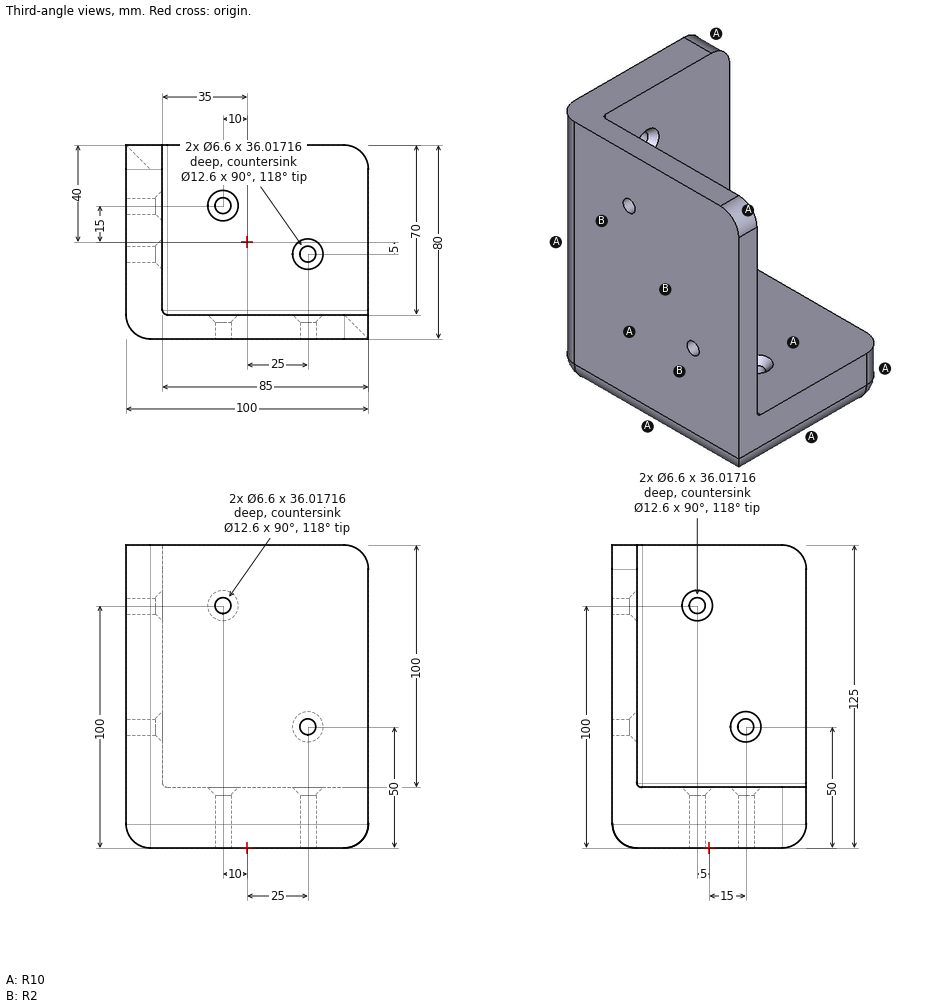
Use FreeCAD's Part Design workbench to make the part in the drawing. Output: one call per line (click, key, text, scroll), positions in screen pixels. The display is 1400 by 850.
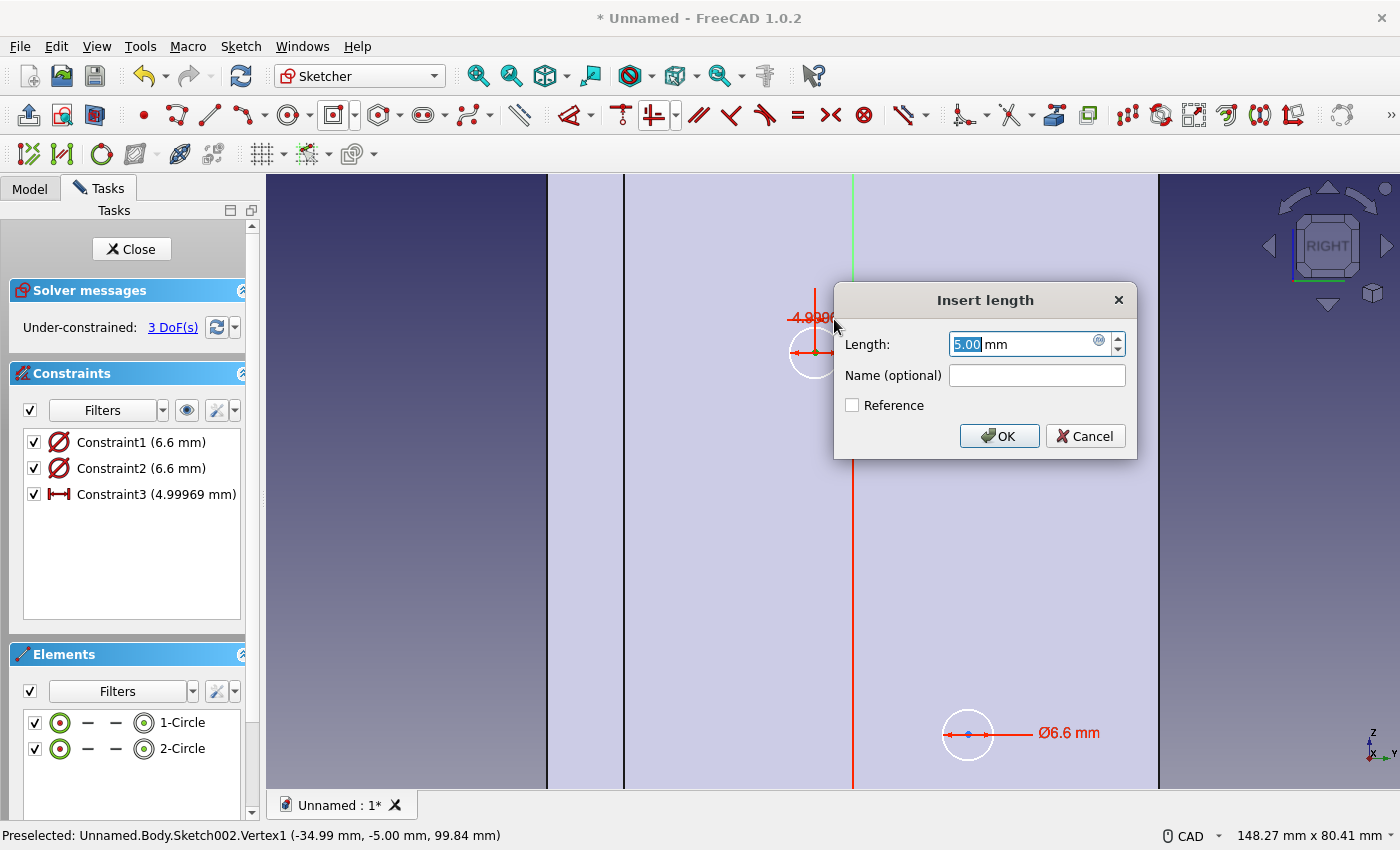
text(5)
key(Return)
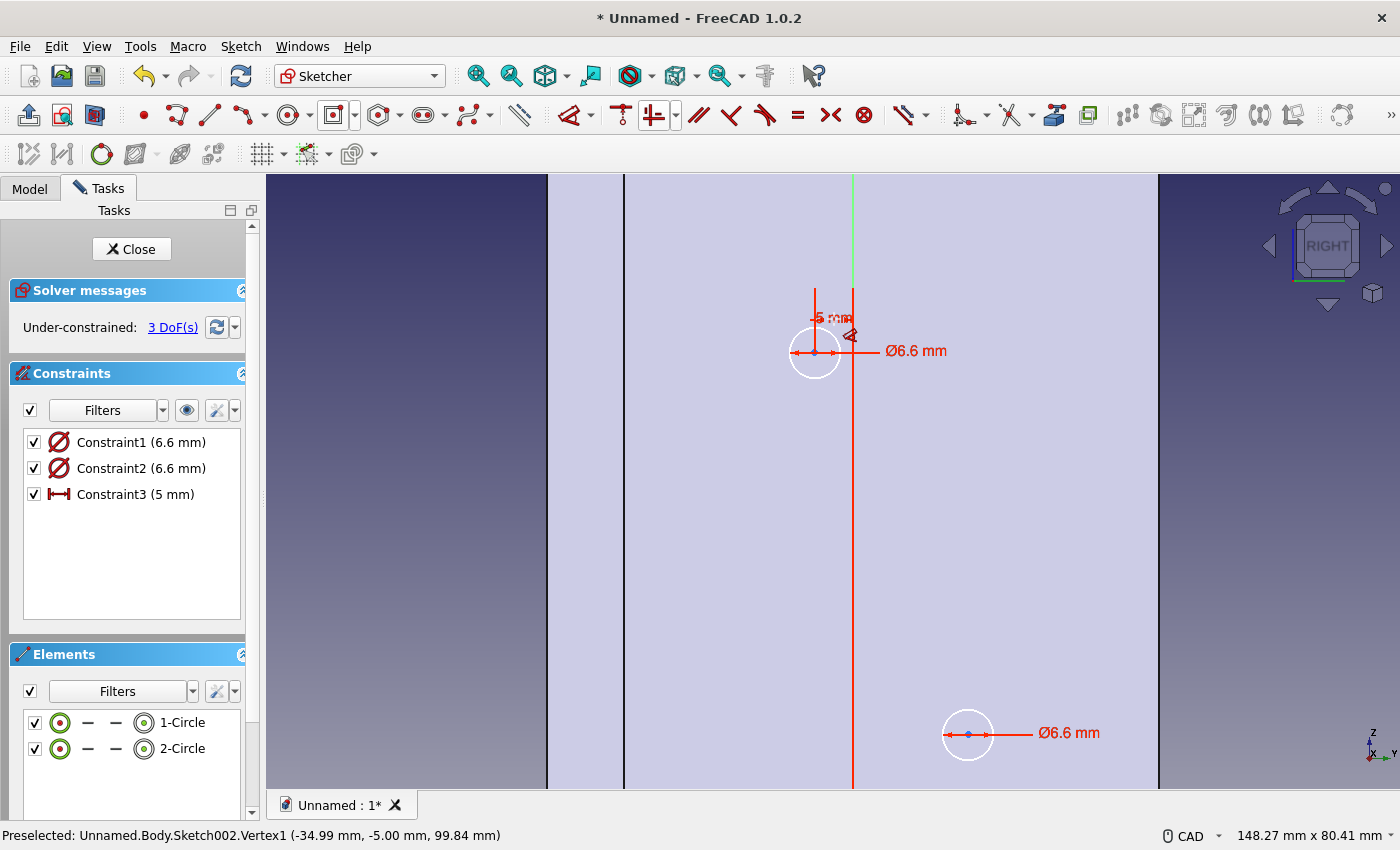
click(968, 735)
click(911, 701)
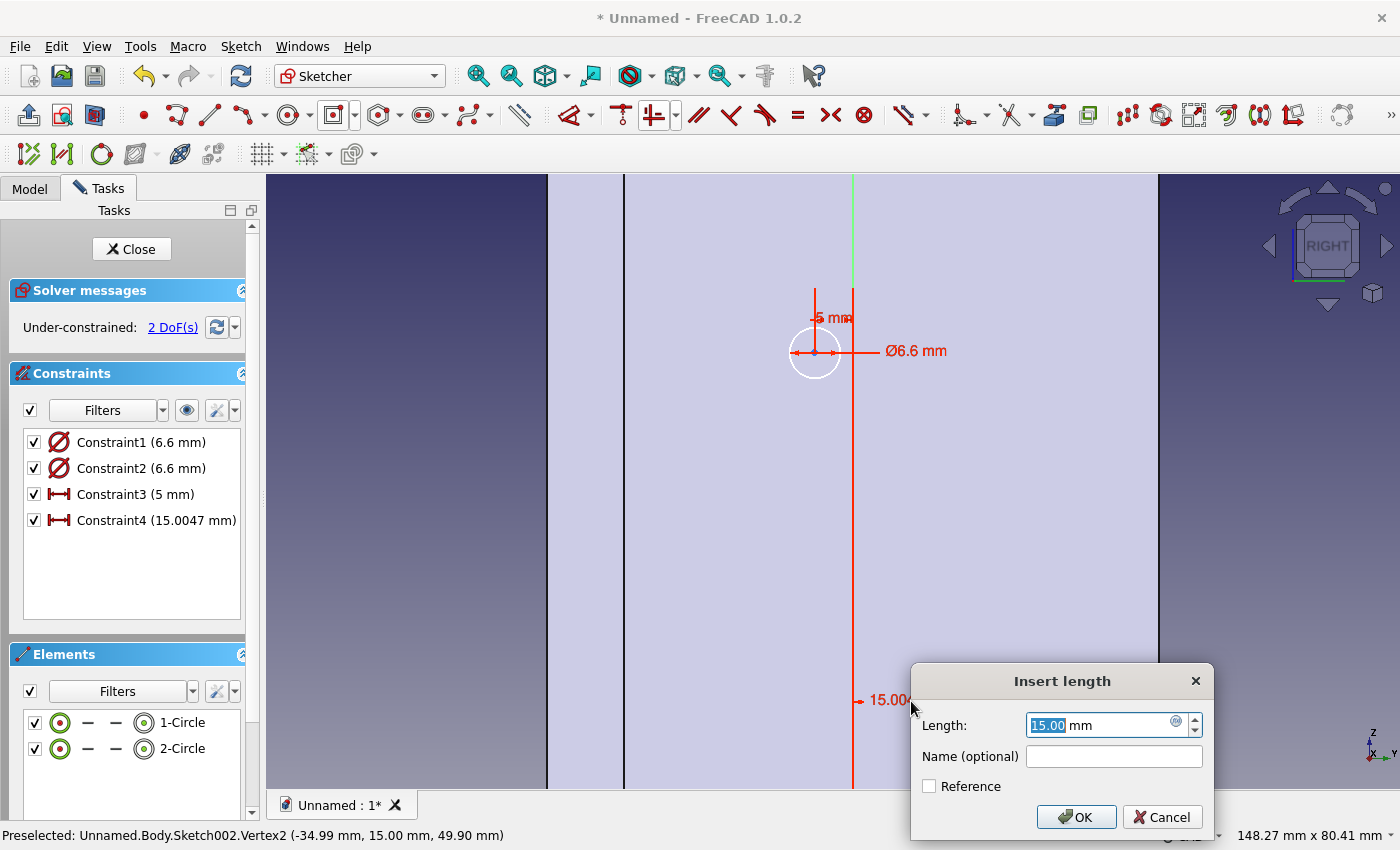
text(15)
key(Return)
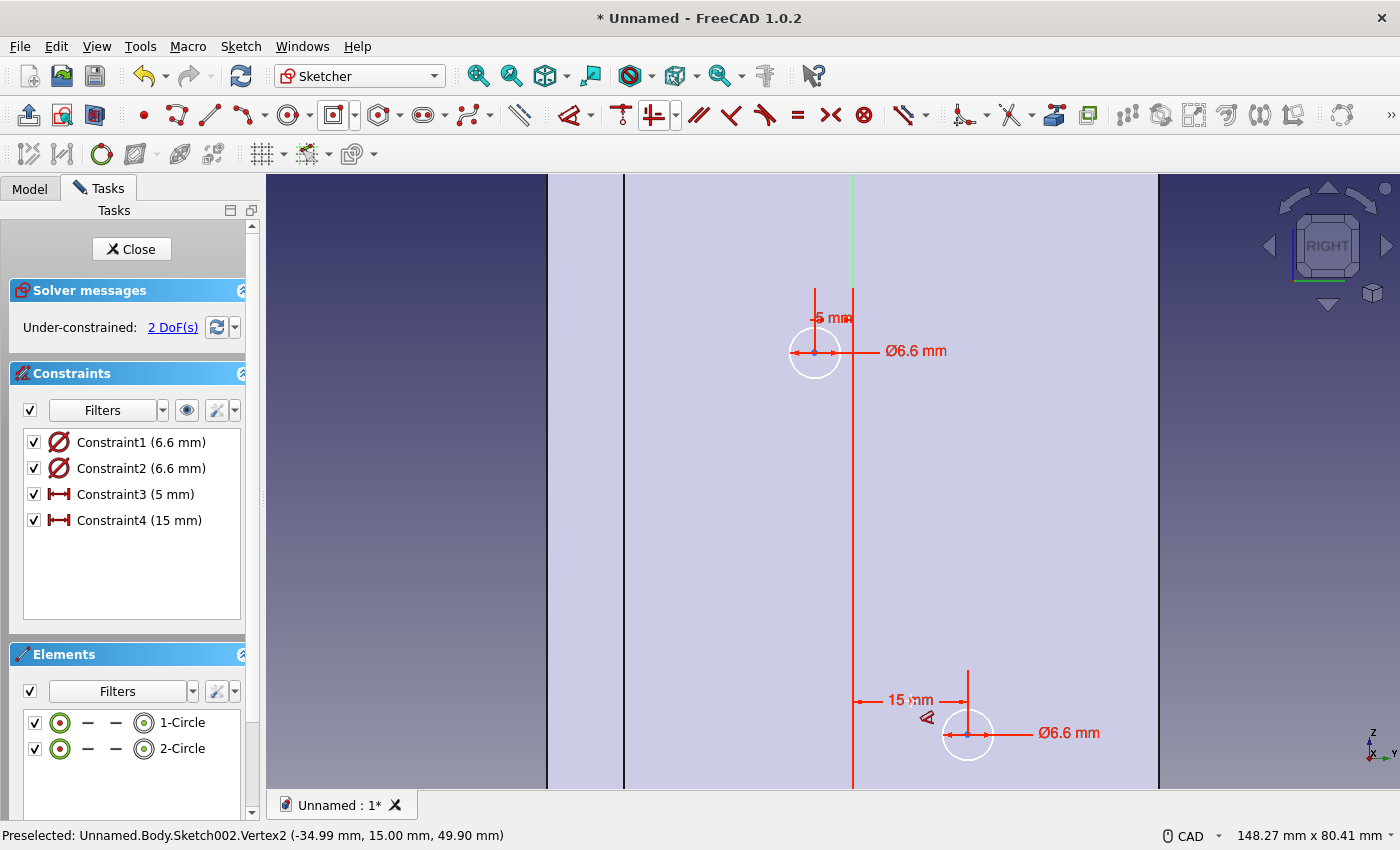
click(968, 735)
click(1002, 754)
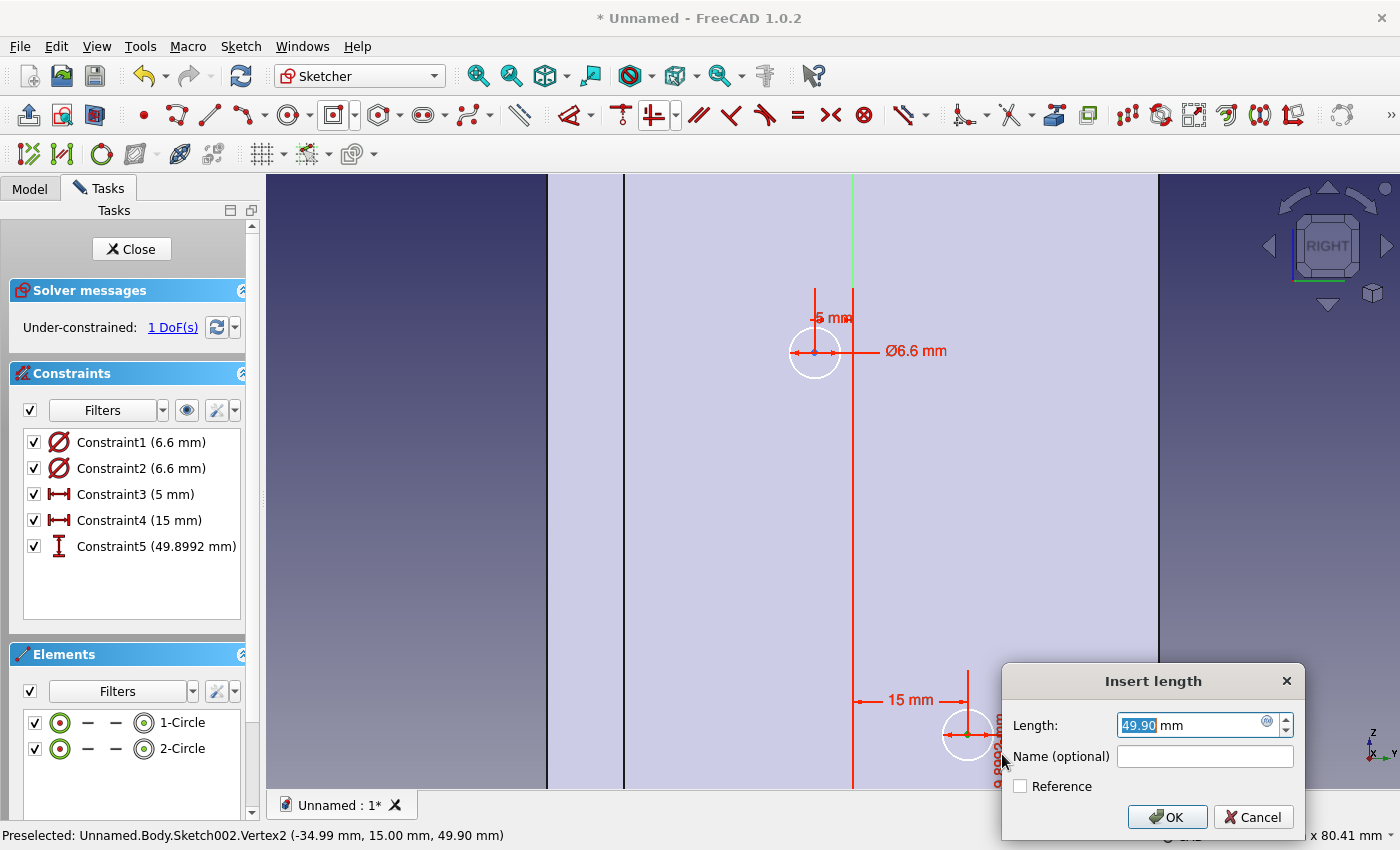
text(50)
key(Return)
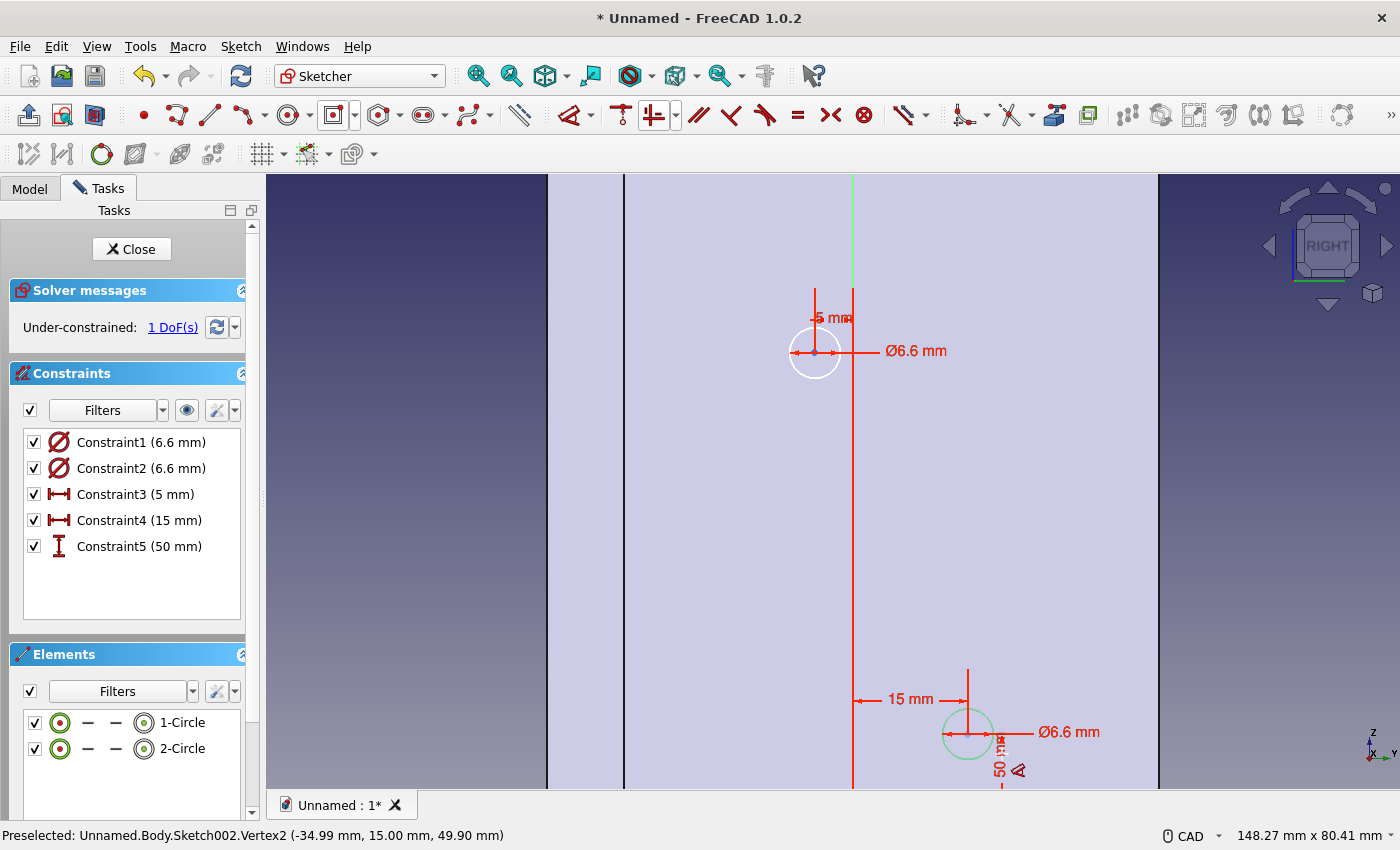
click(815, 353)
click(781, 557)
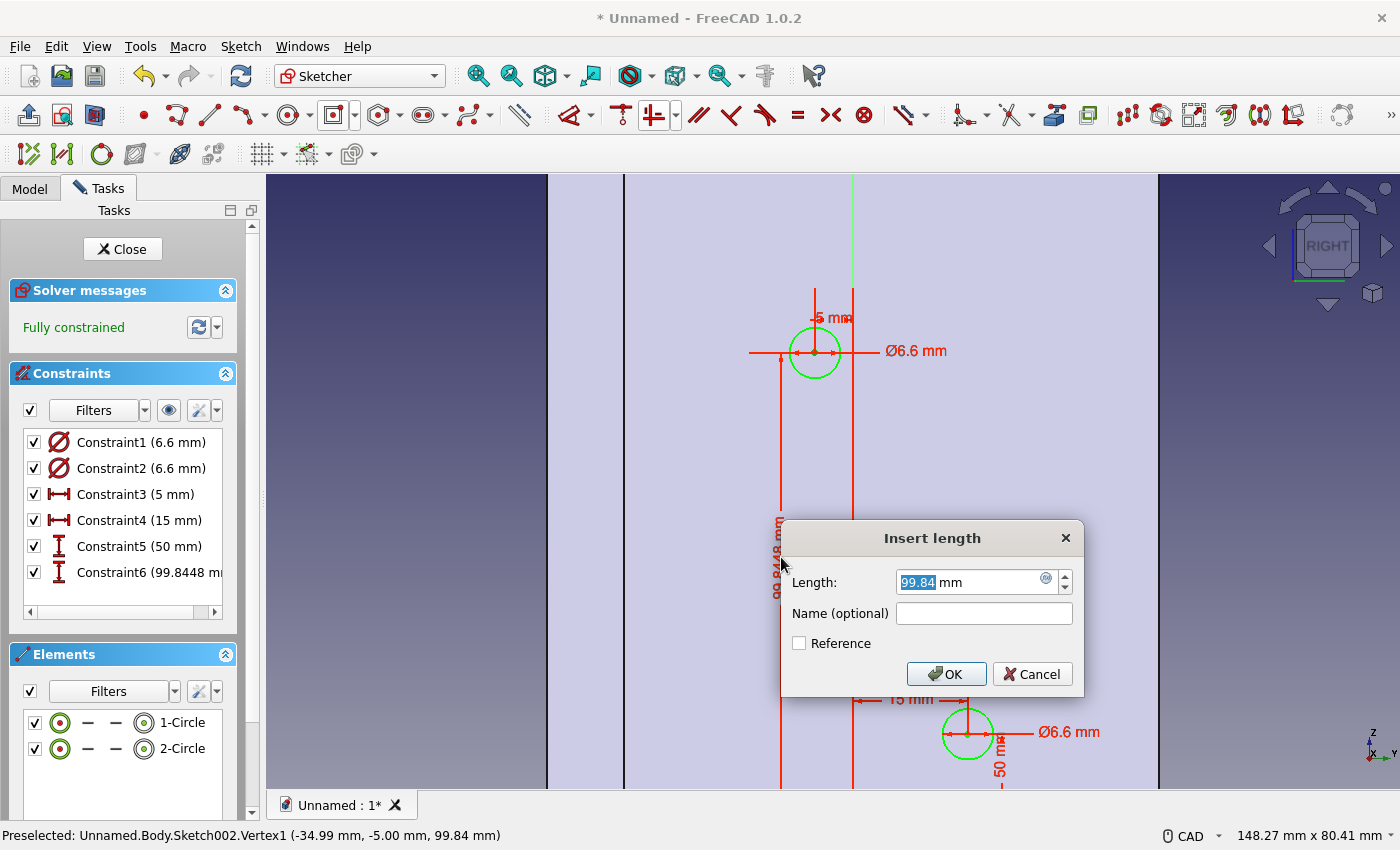
text(100)
key(Return)
key(Escape)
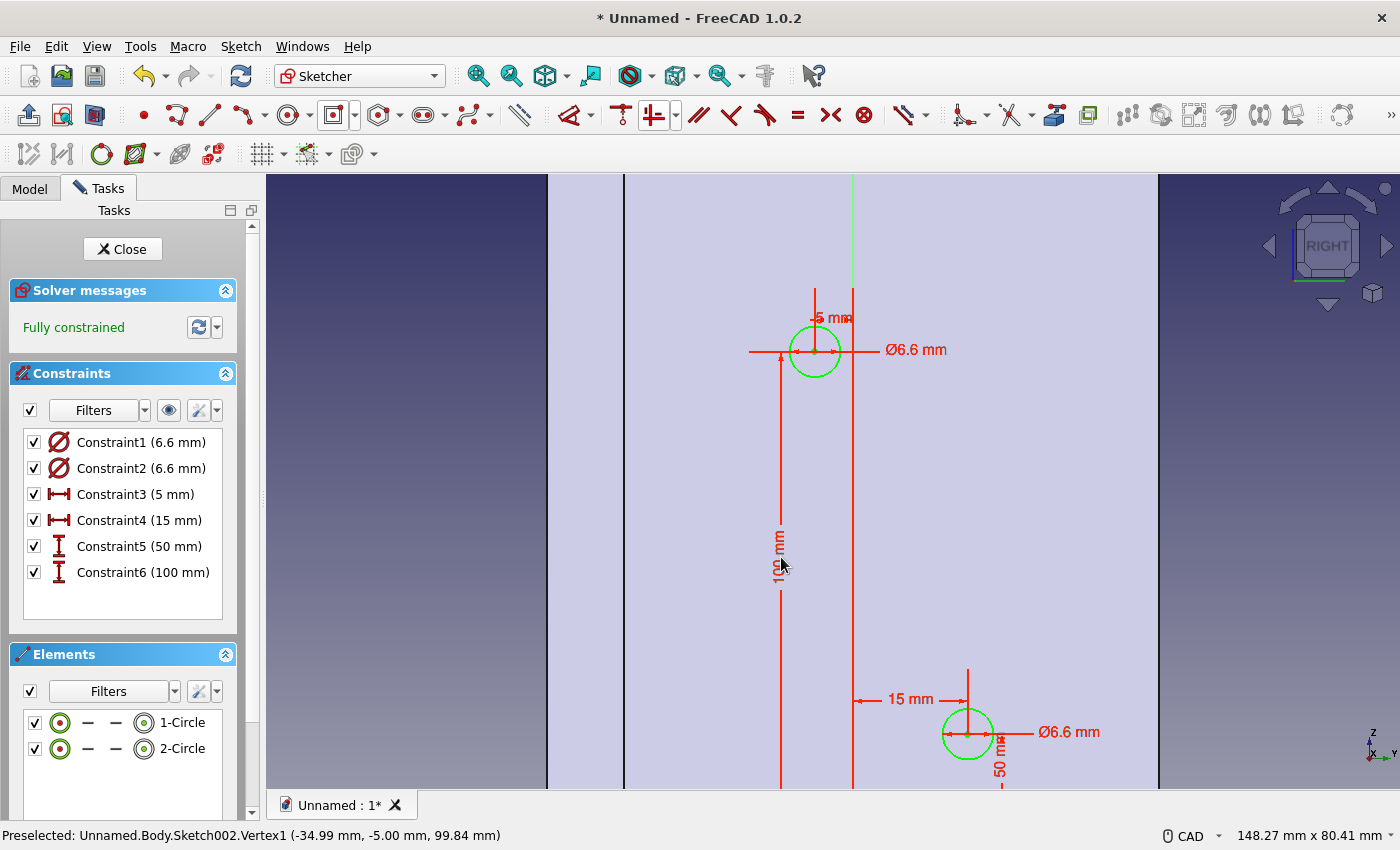
click(123, 249)